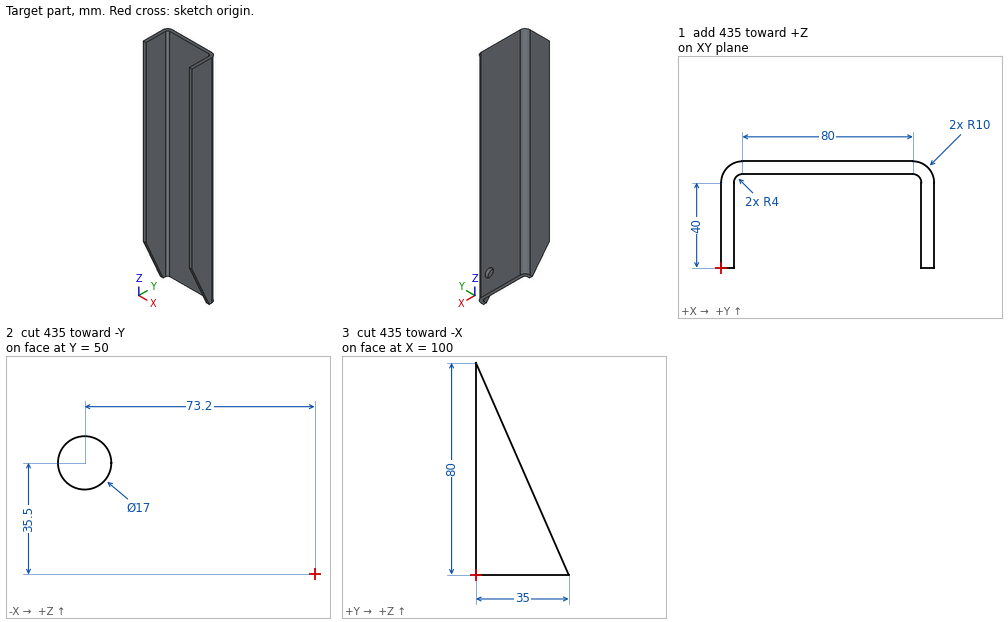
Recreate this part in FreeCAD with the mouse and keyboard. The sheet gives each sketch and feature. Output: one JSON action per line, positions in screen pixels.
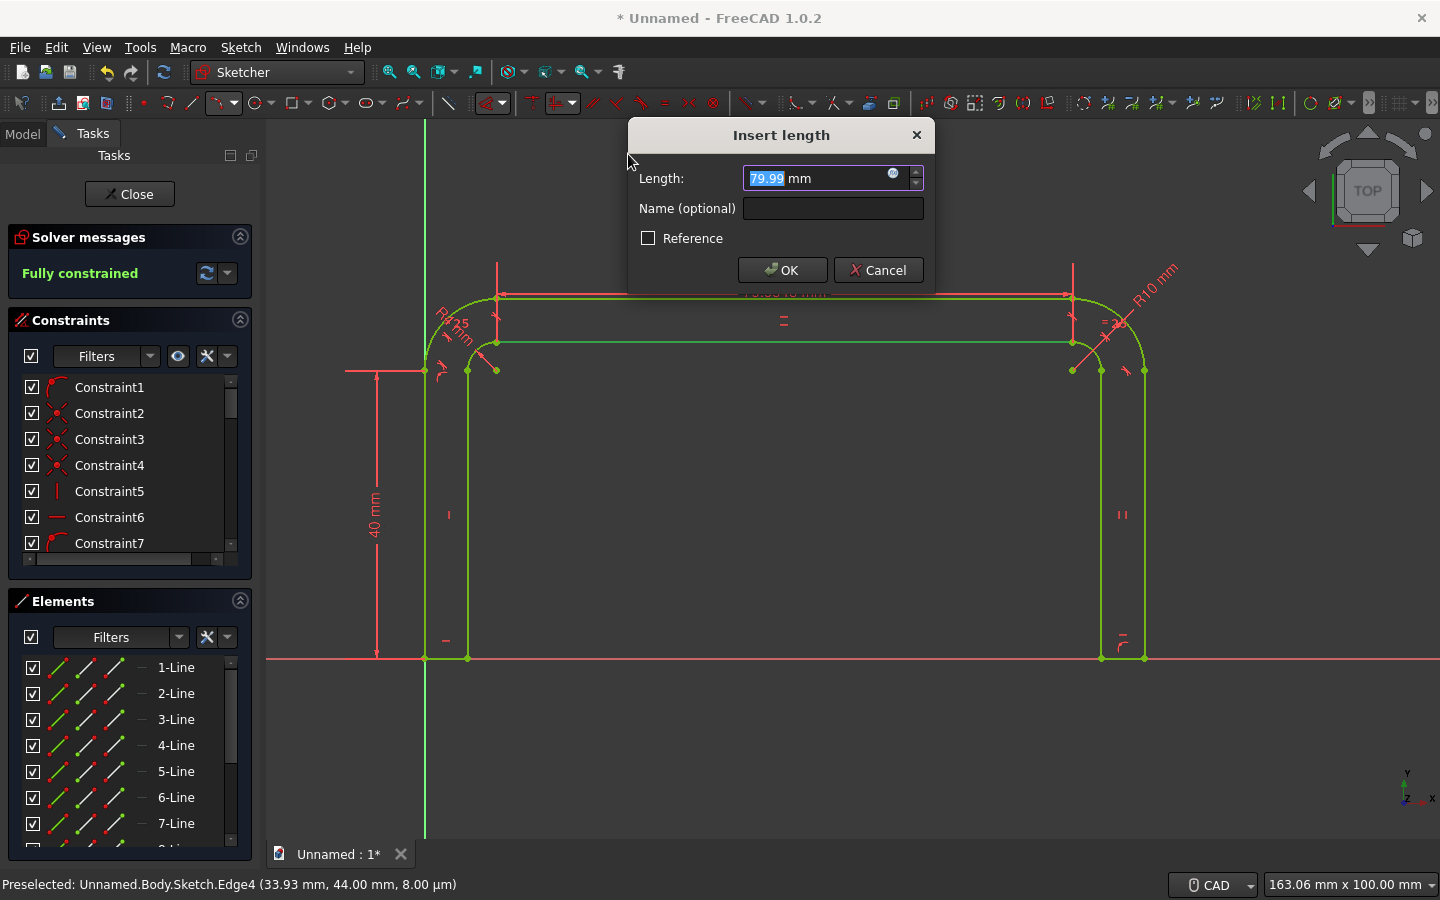
{"action": "type", "text": "80"}
{"action": "key", "text": "Return"}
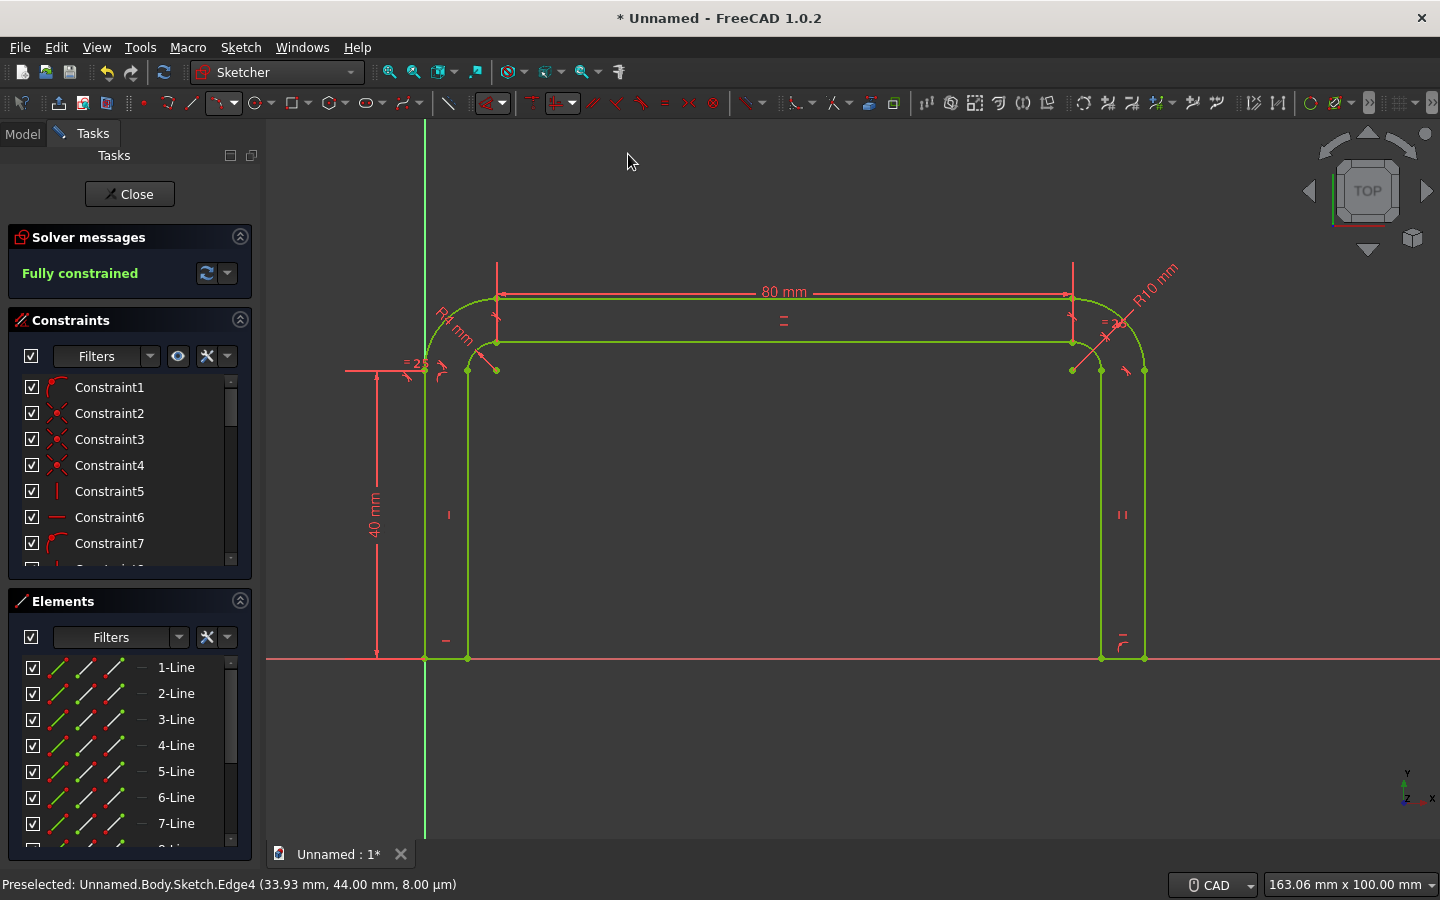
{"action": "left_click", "coordinate": [130, 194]}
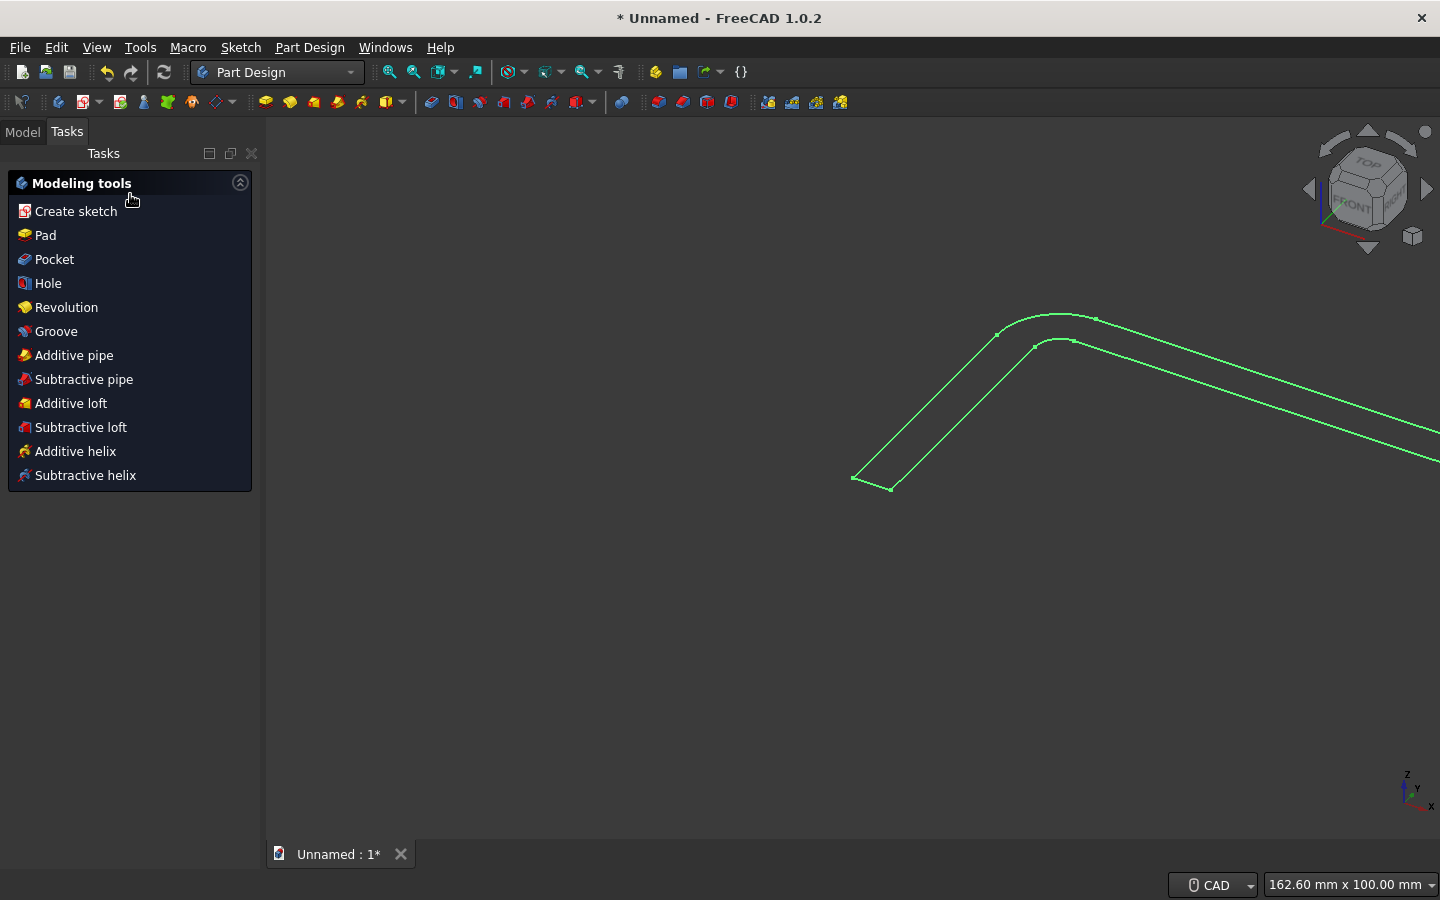
{"action": "left_click", "coordinate": [266, 102]}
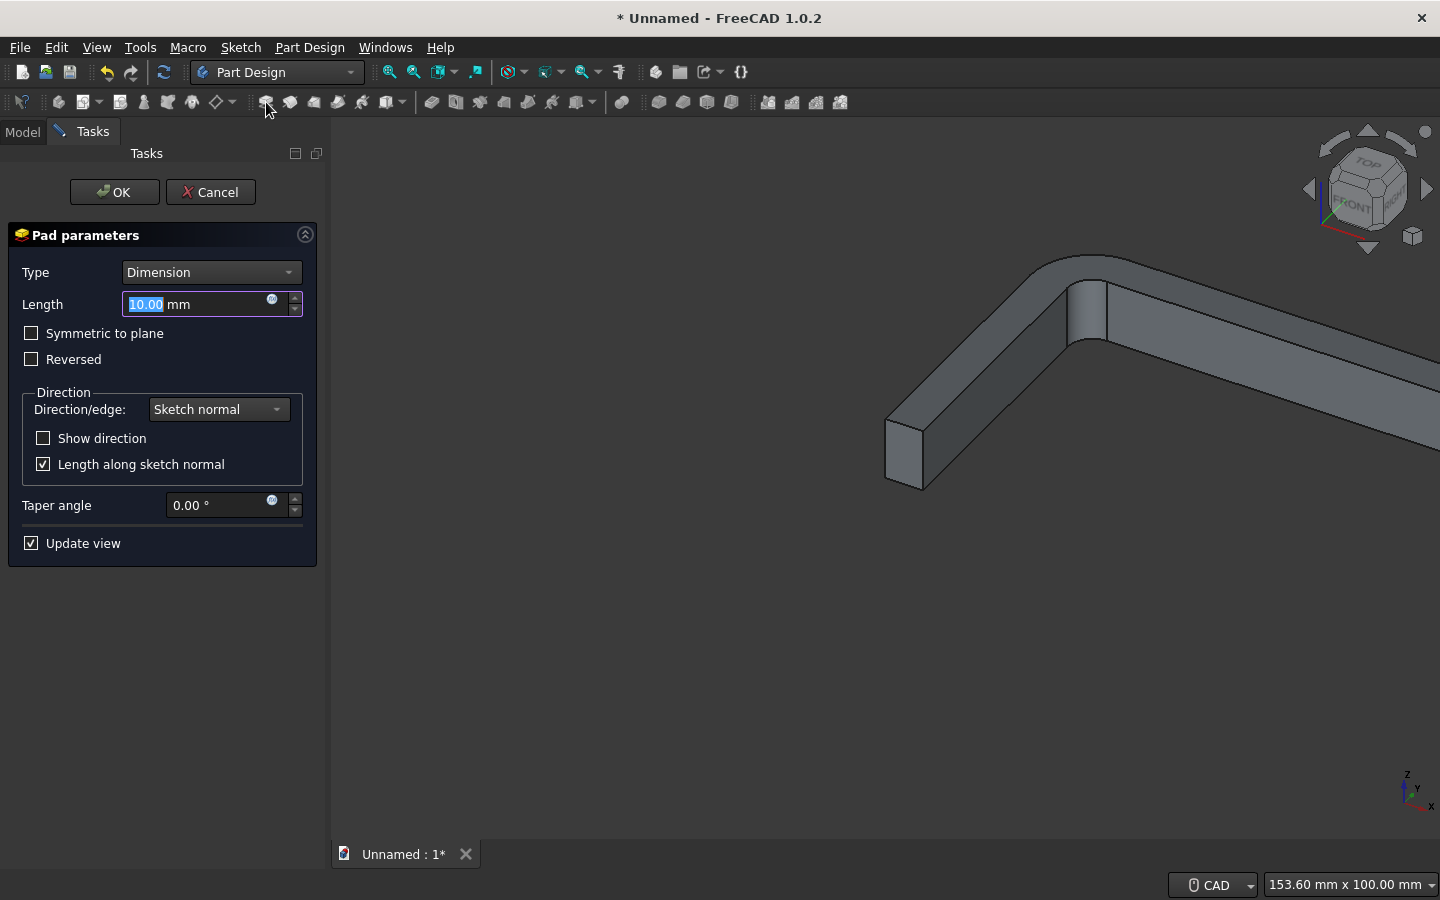
{"action": "type", "text": "435"}
{"action": "key", "text": "Tab"}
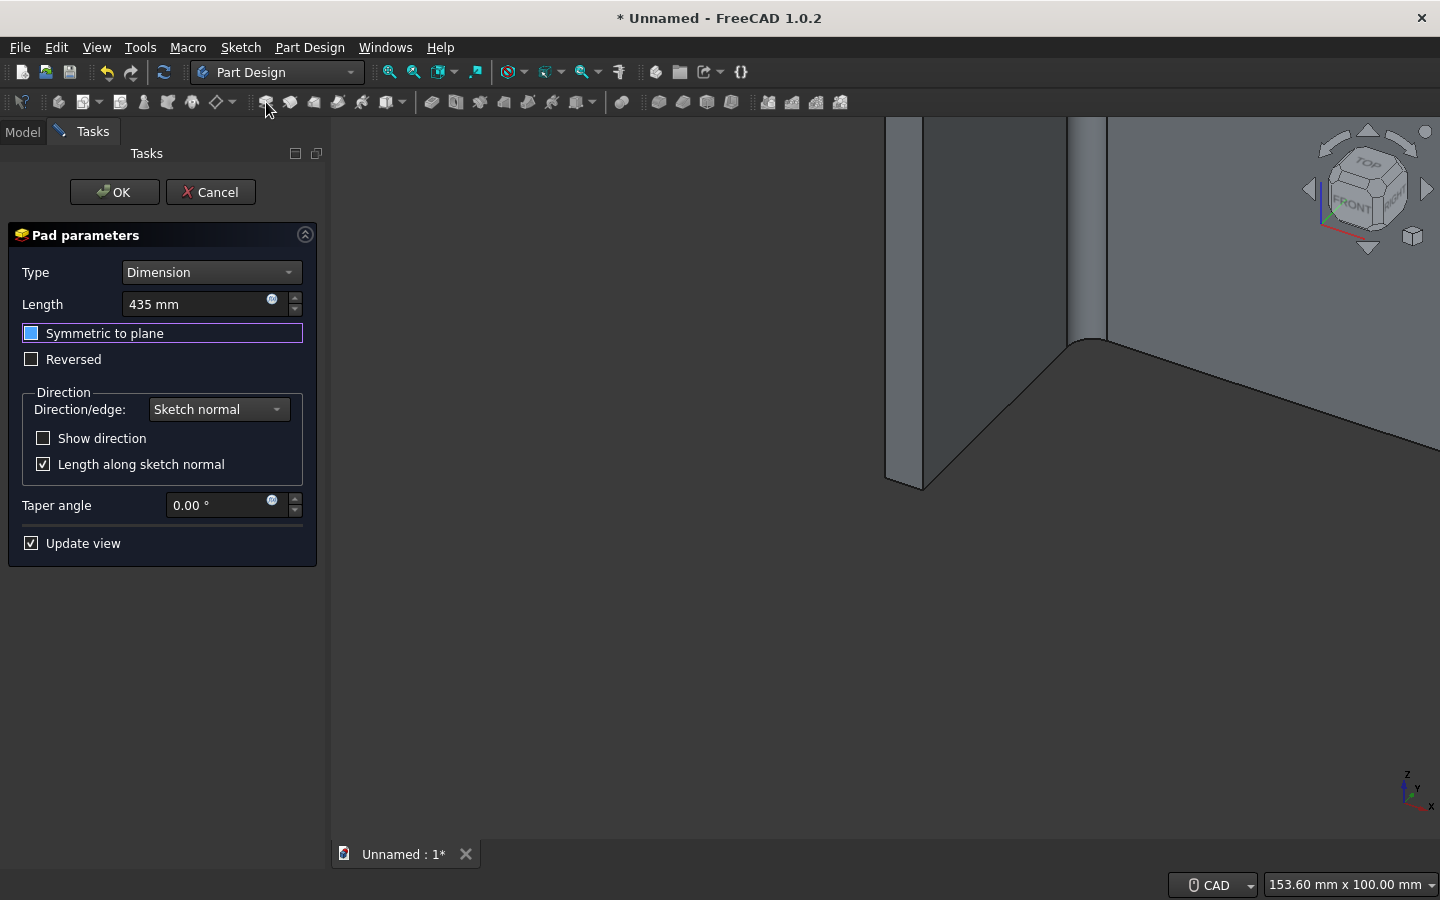
{"action": "left_click", "coordinate": [115, 192]}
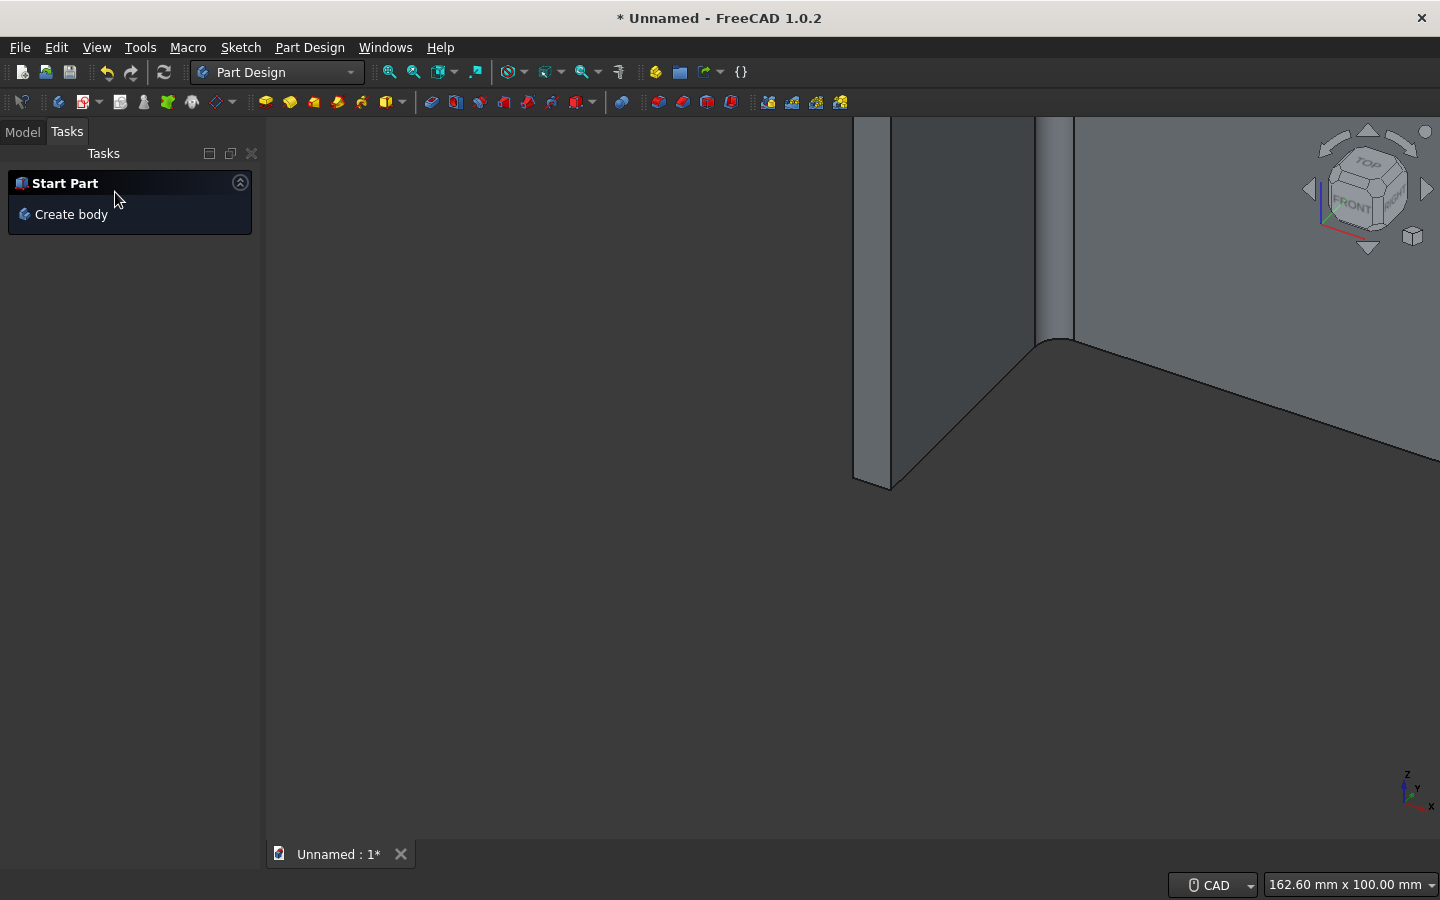
{"action": "left_click", "coordinate": [390, 72]}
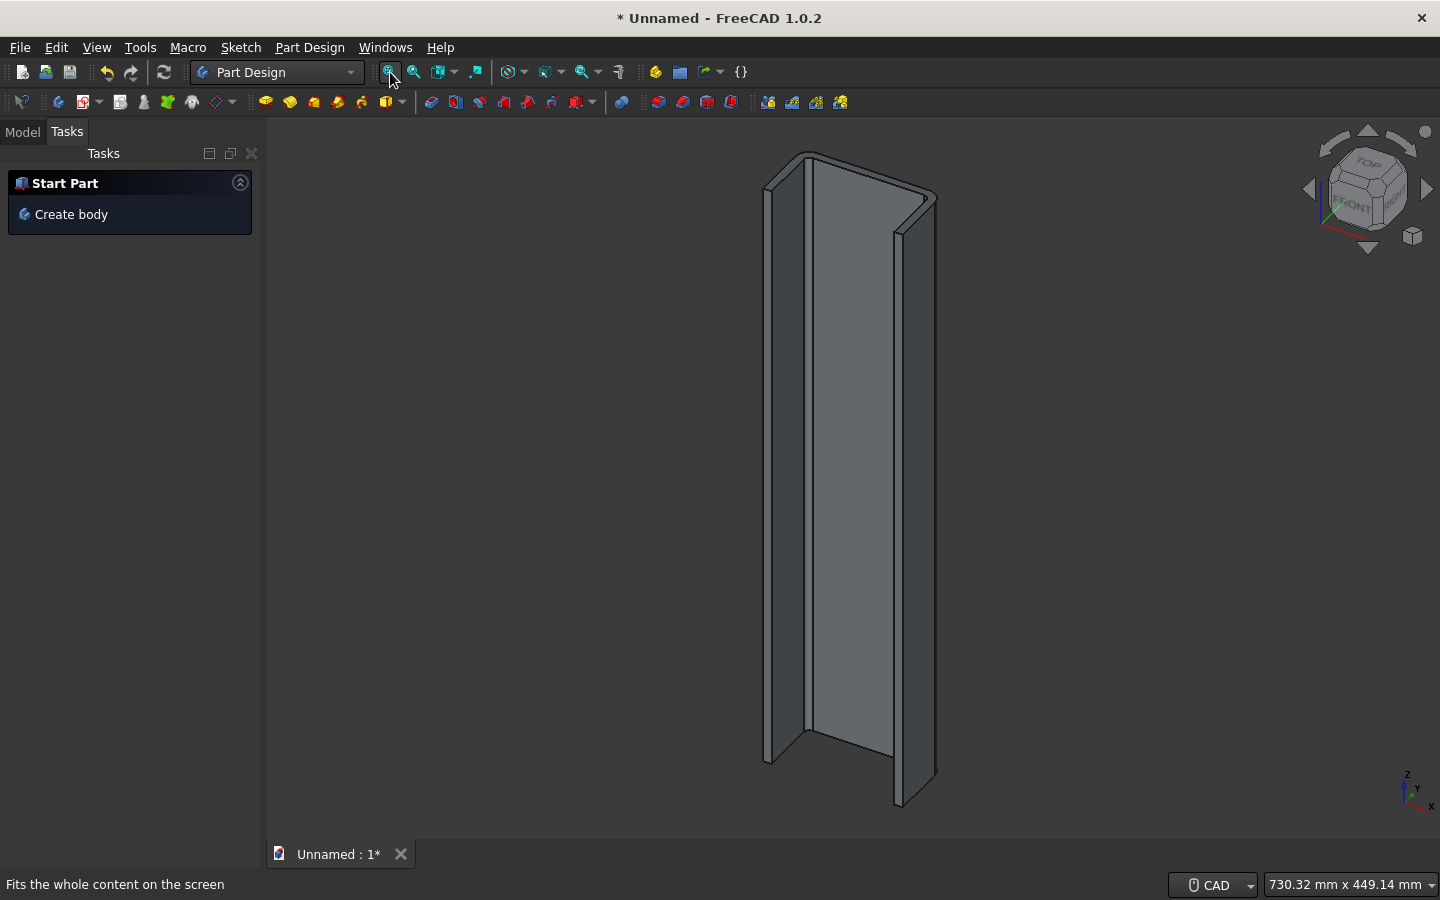
{"action": "key", "text": "4"}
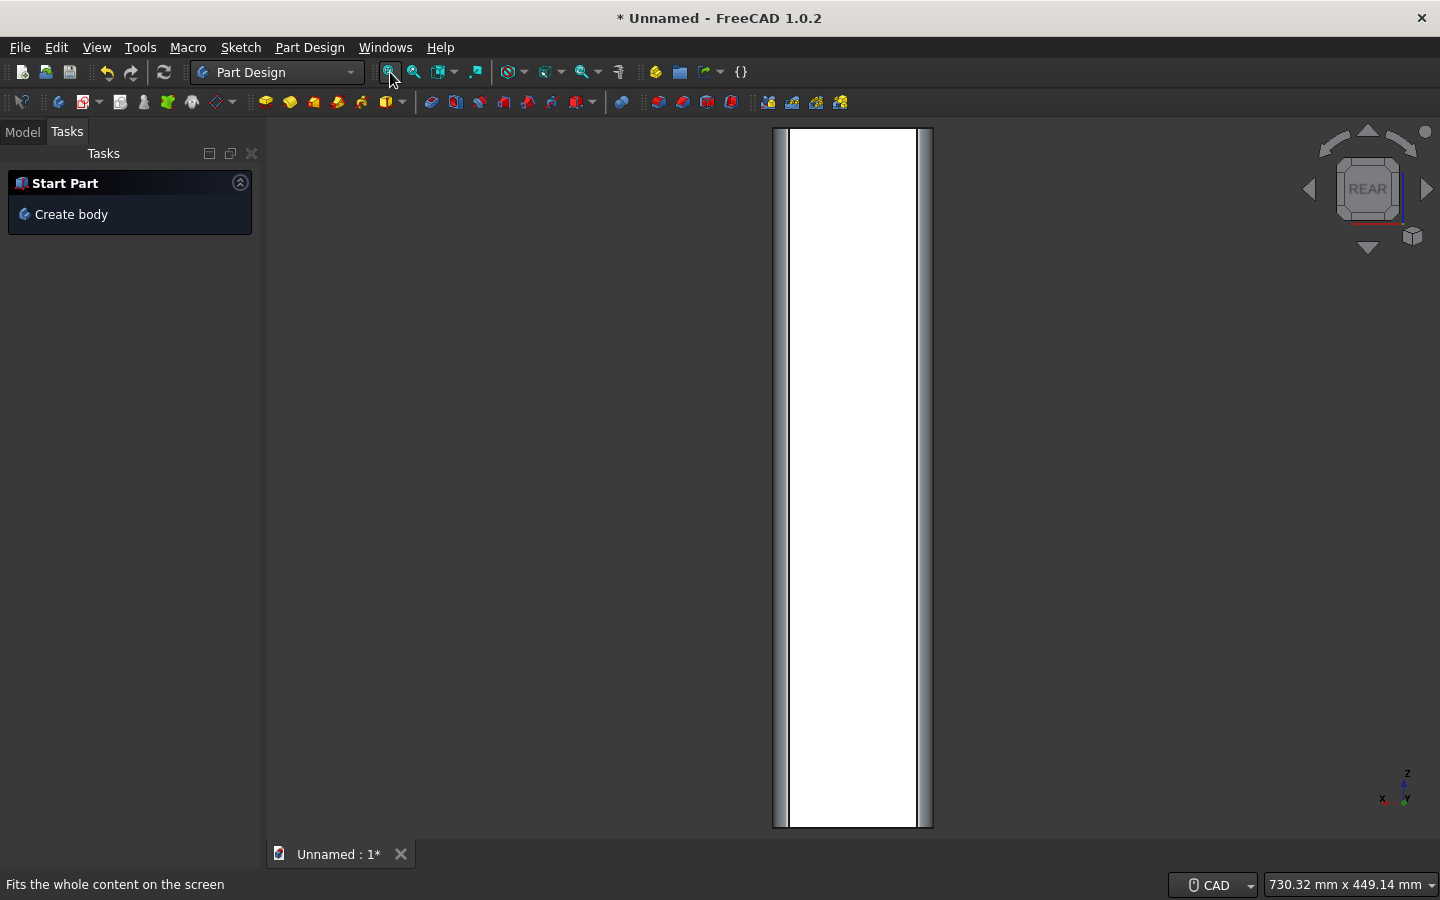
{"action": "left_click", "coordinate": [853, 277]}